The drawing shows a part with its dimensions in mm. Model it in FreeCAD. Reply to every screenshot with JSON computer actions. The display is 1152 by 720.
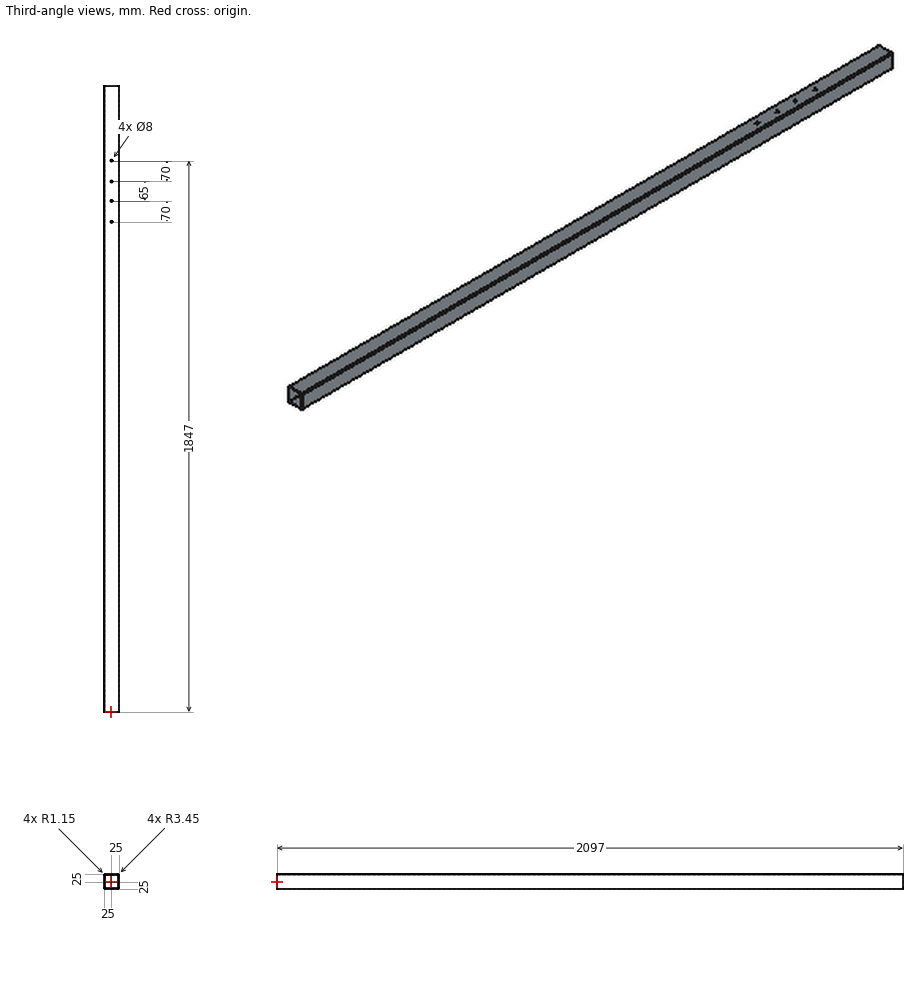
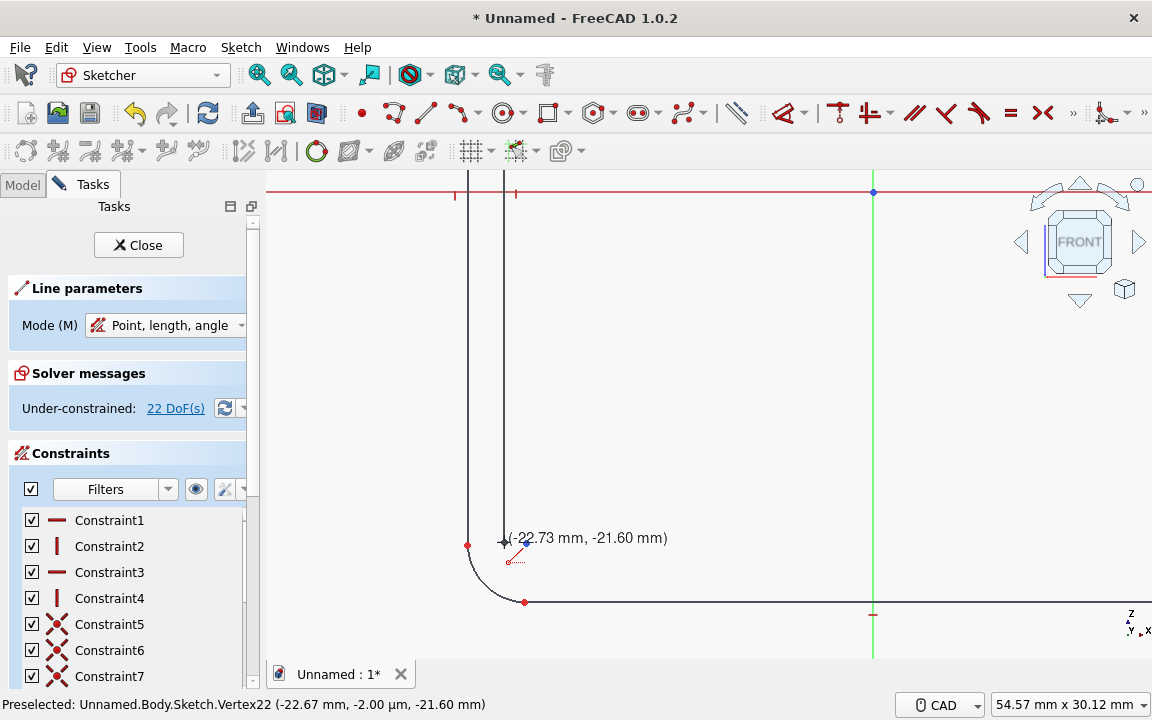
{"action": "left_click", "coordinate": [523, 561]}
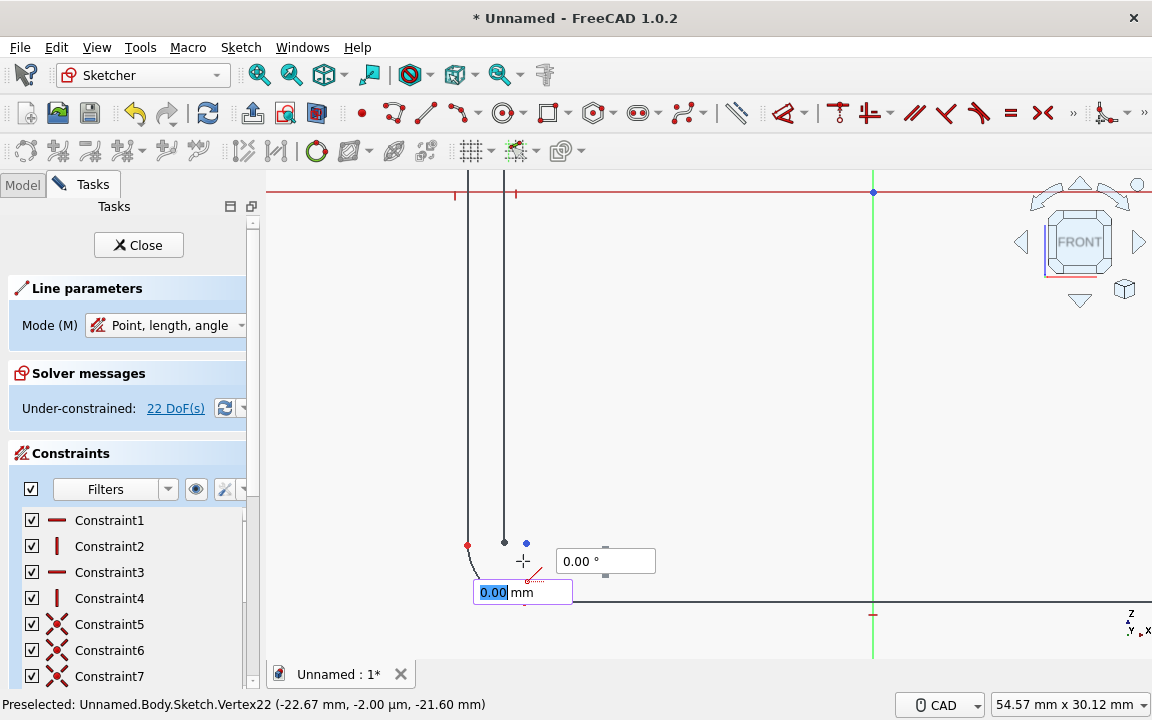
{"action": "scroll", "coordinate": [505, 544], "scroll_direction": "down", "scroll_amount": 5}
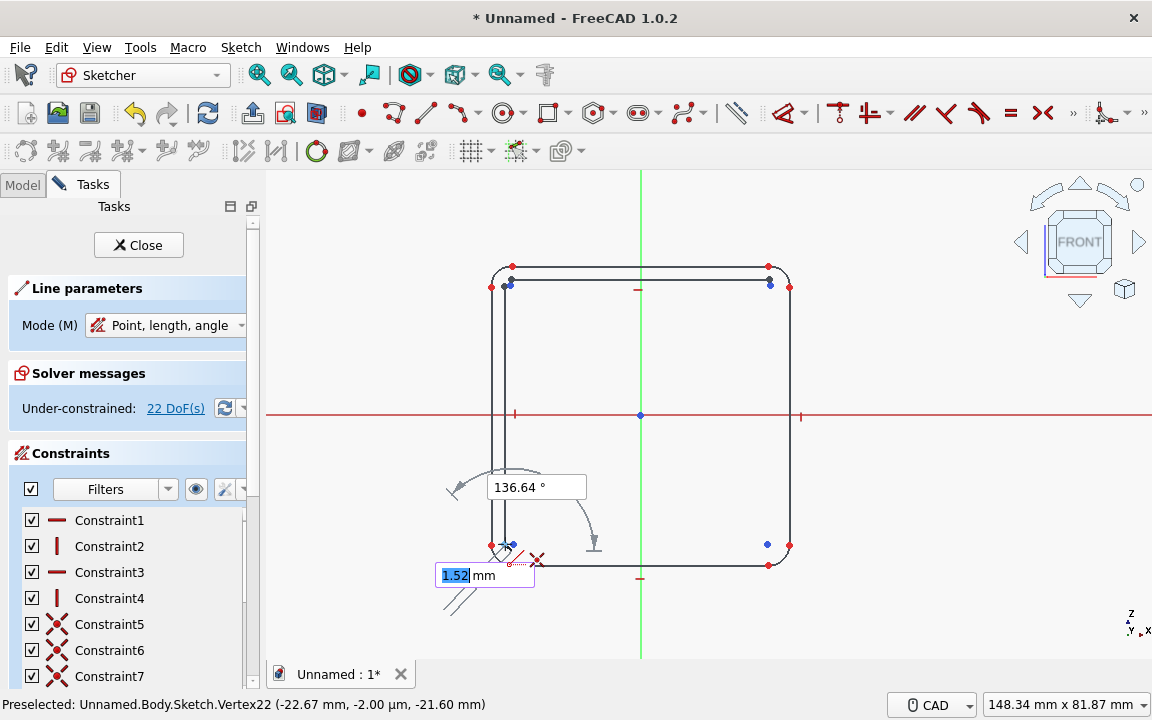
{"action": "scroll", "coordinate": [769, 551], "scroll_direction": "up", "scroll_amount": 5}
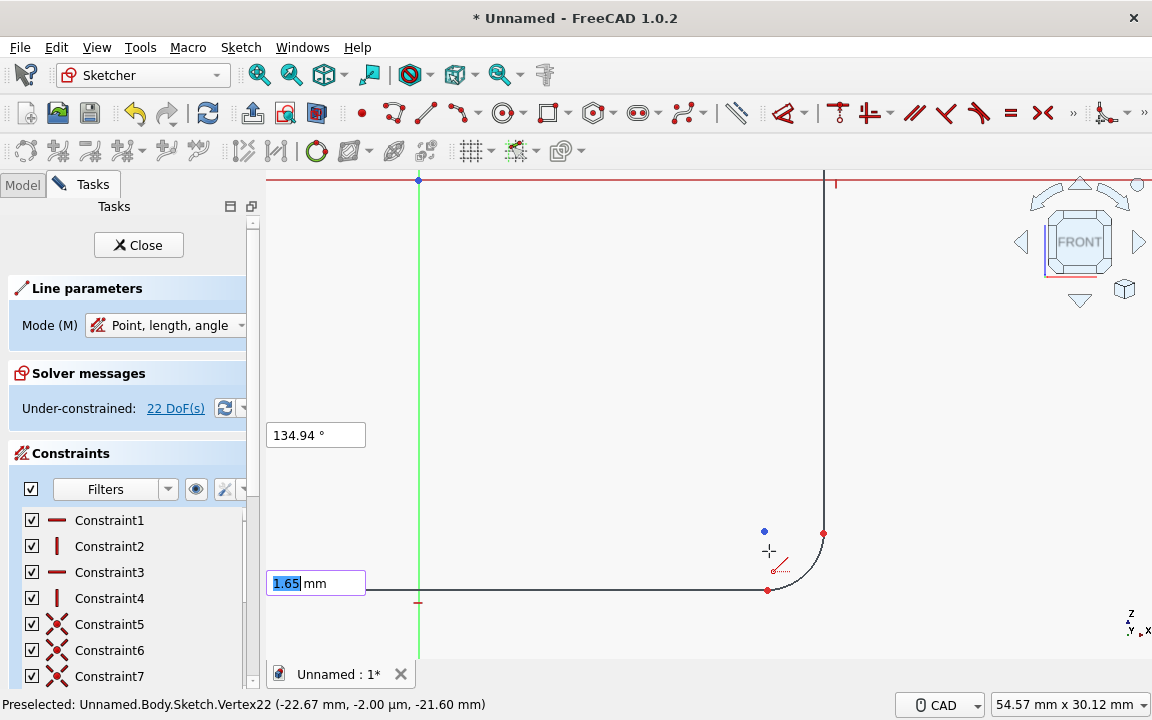
{"action": "left_click", "coordinate": [769, 549]}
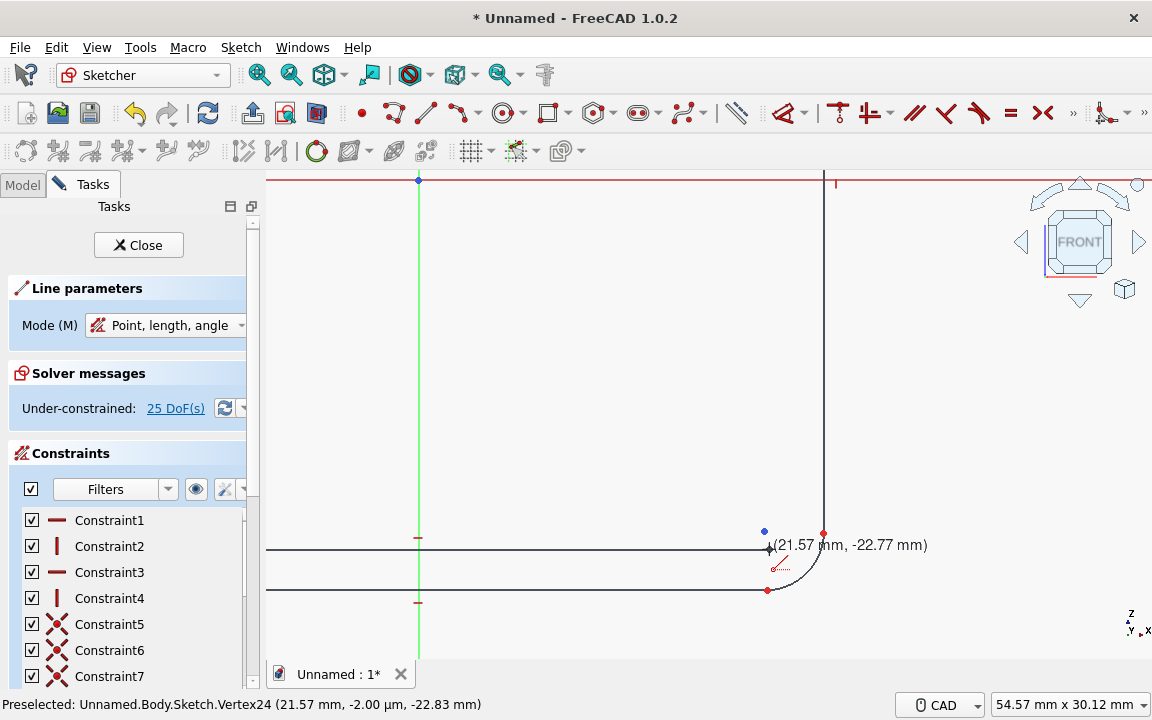
{"action": "left_click", "coordinate": [787, 530]}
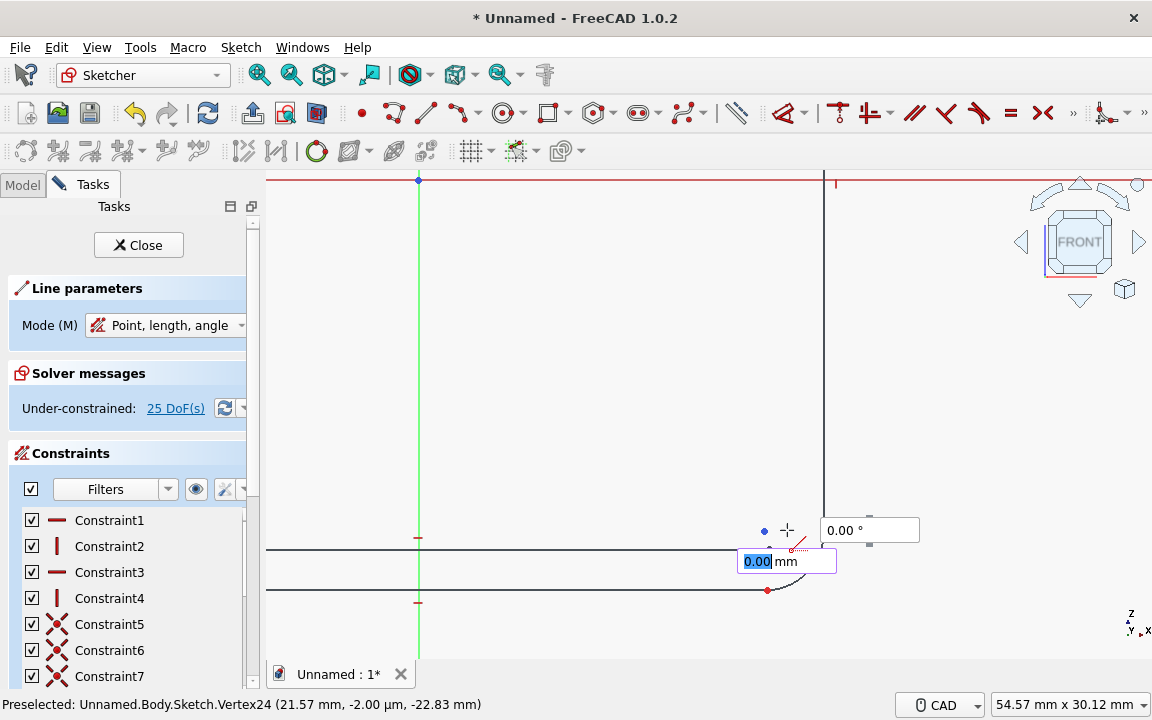
{"action": "scroll", "coordinate": [769, 551], "scroll_direction": "down", "scroll_amount": 5}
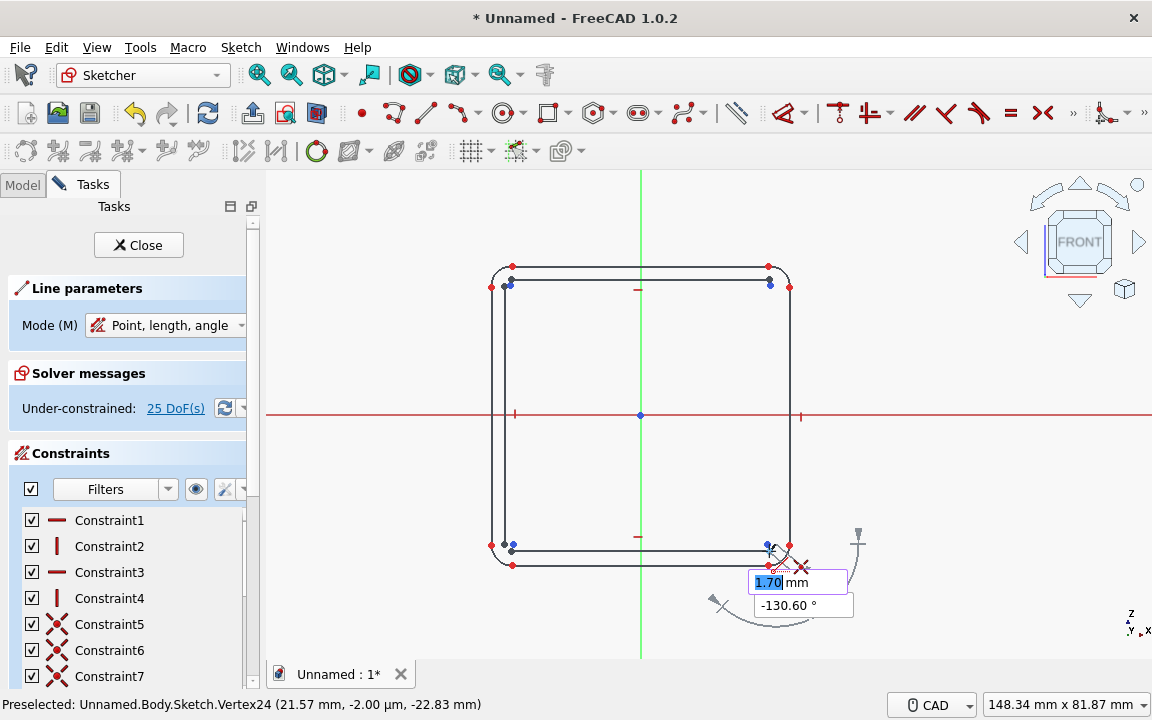
{"action": "scroll", "coordinate": [776, 286], "scroll_direction": "up", "scroll_amount": 5}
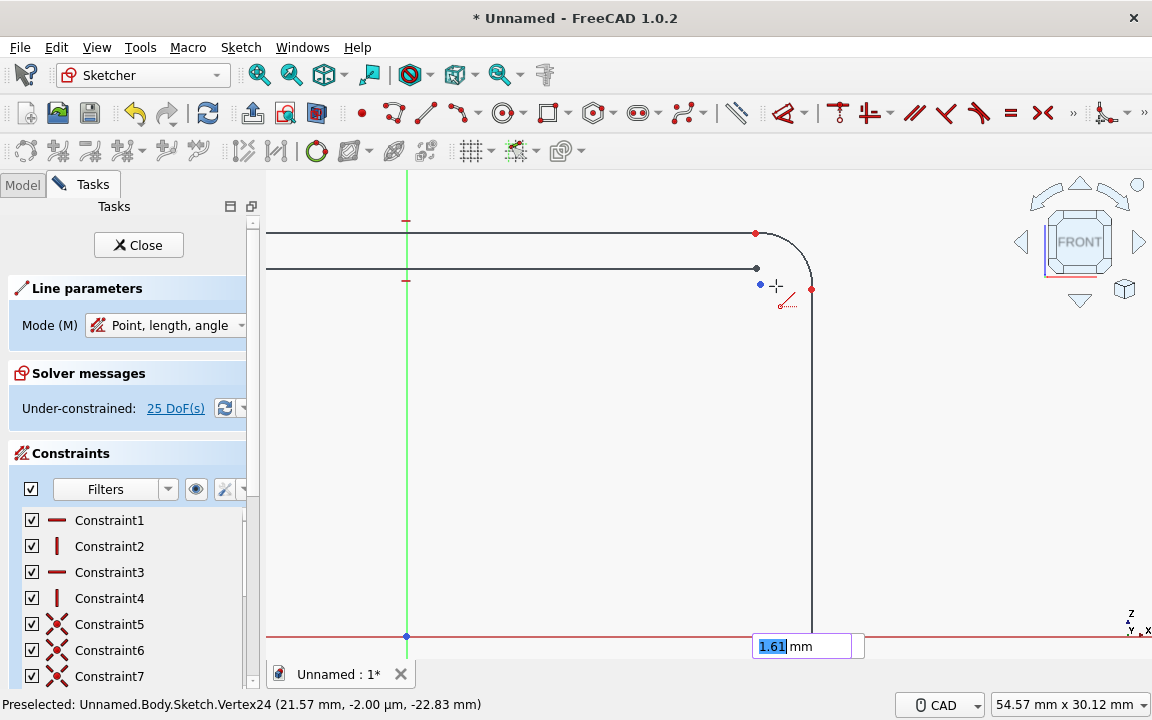
{"action": "left_click", "coordinate": [775, 287]}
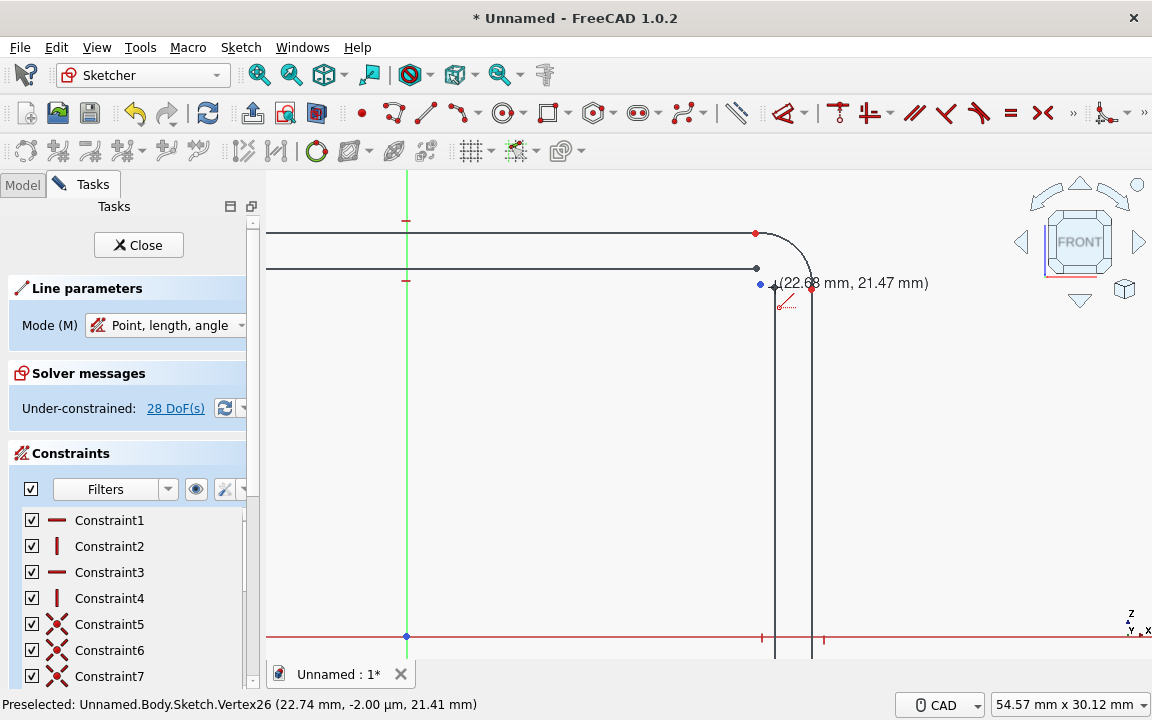
{"action": "left_click", "coordinate": [458, 114]}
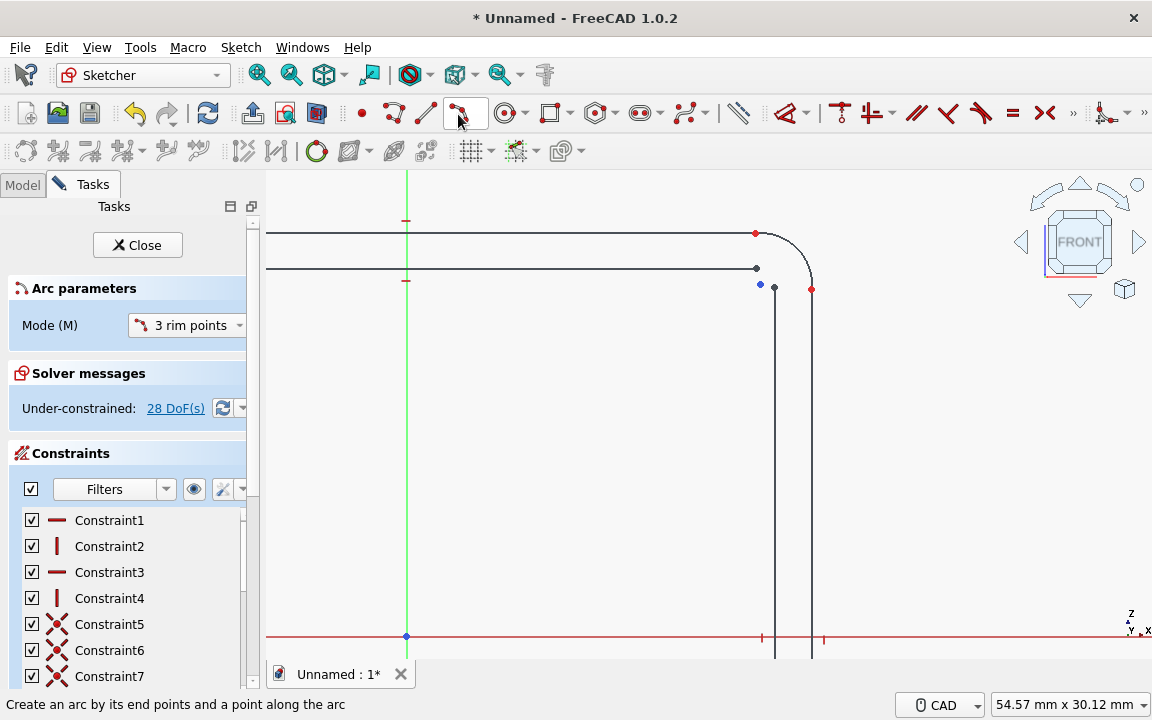
{"action": "scroll", "coordinate": [776, 285], "scroll_direction": "down", "scroll_amount": 5}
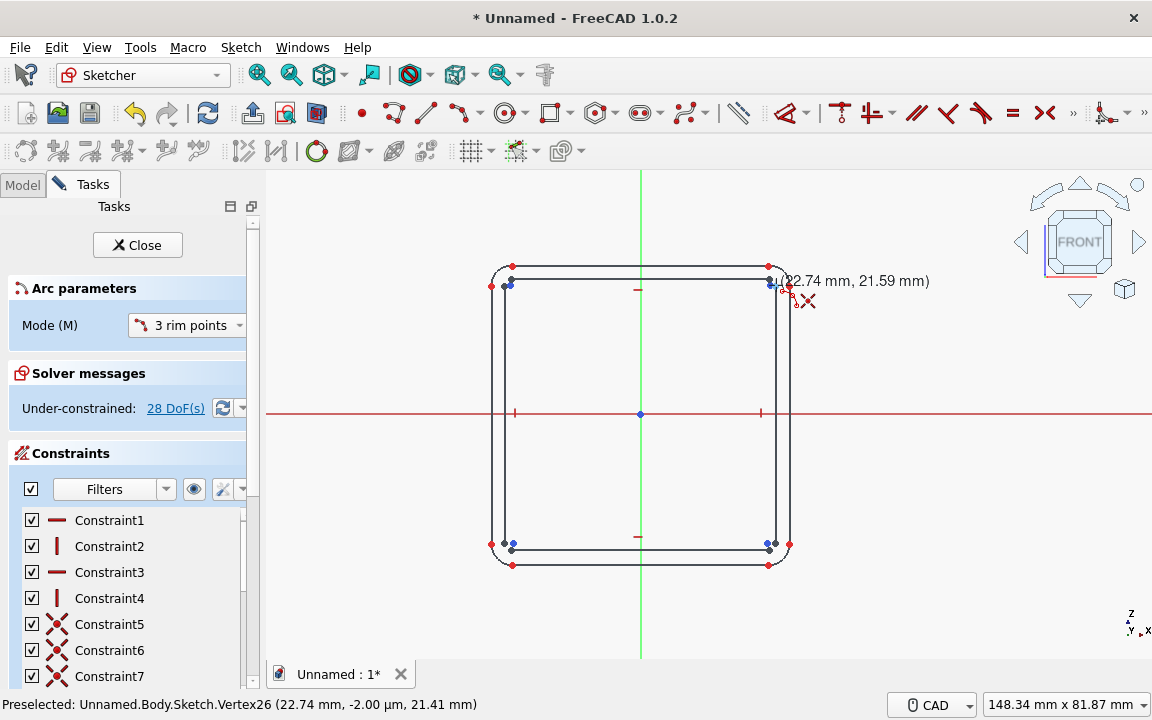
{"action": "scroll", "coordinate": [512, 279], "scroll_direction": "up", "scroll_amount": 5}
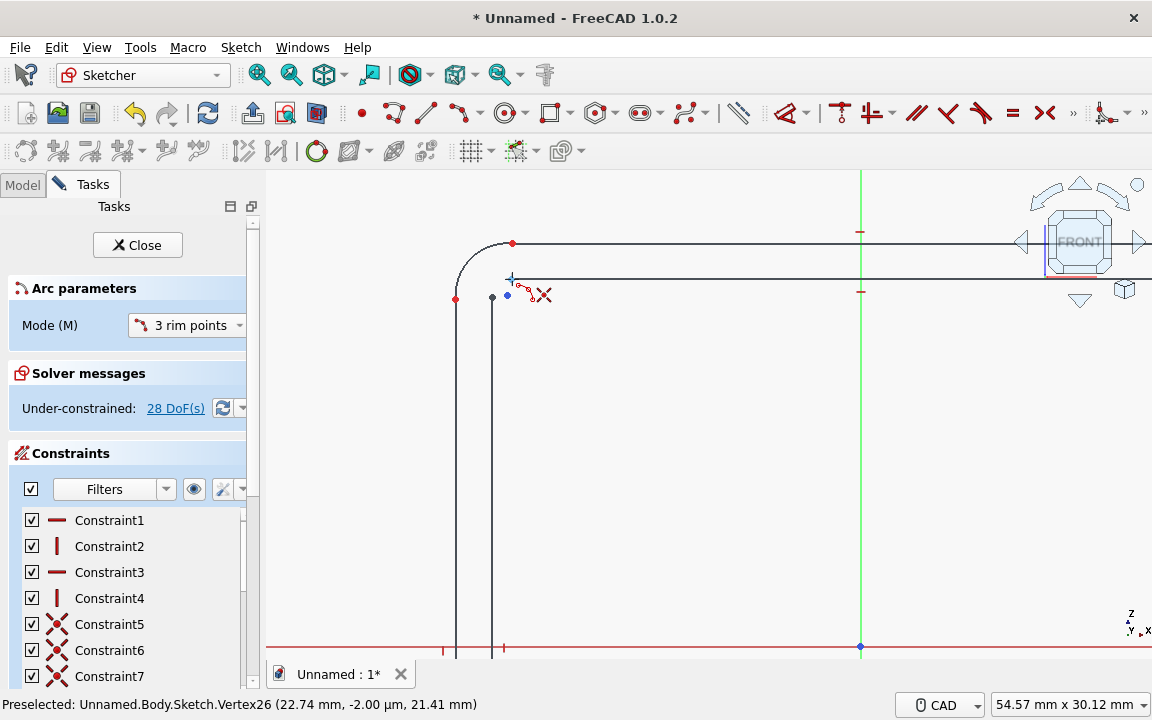
{"action": "left_click", "coordinate": [511, 279]}
{"action": "left_click", "coordinate": [492, 298]}